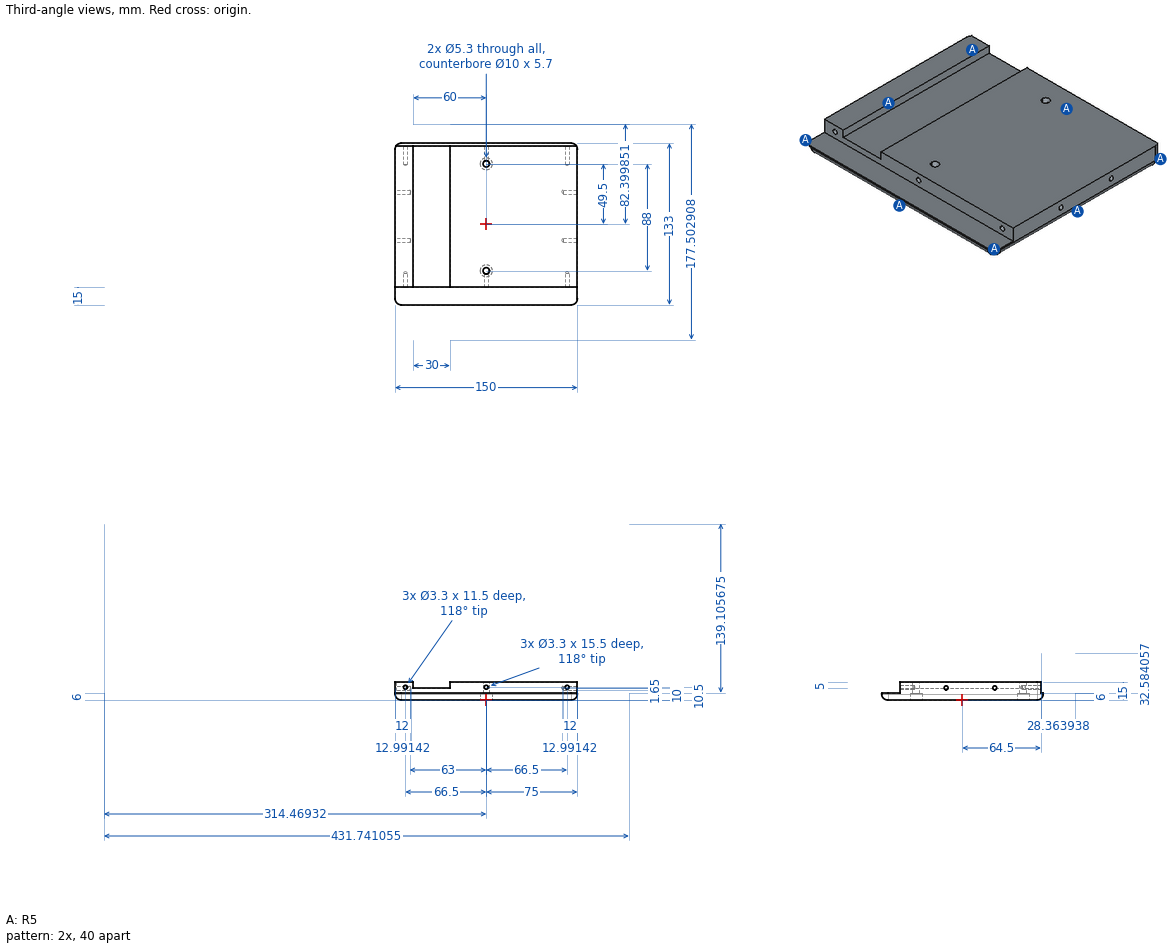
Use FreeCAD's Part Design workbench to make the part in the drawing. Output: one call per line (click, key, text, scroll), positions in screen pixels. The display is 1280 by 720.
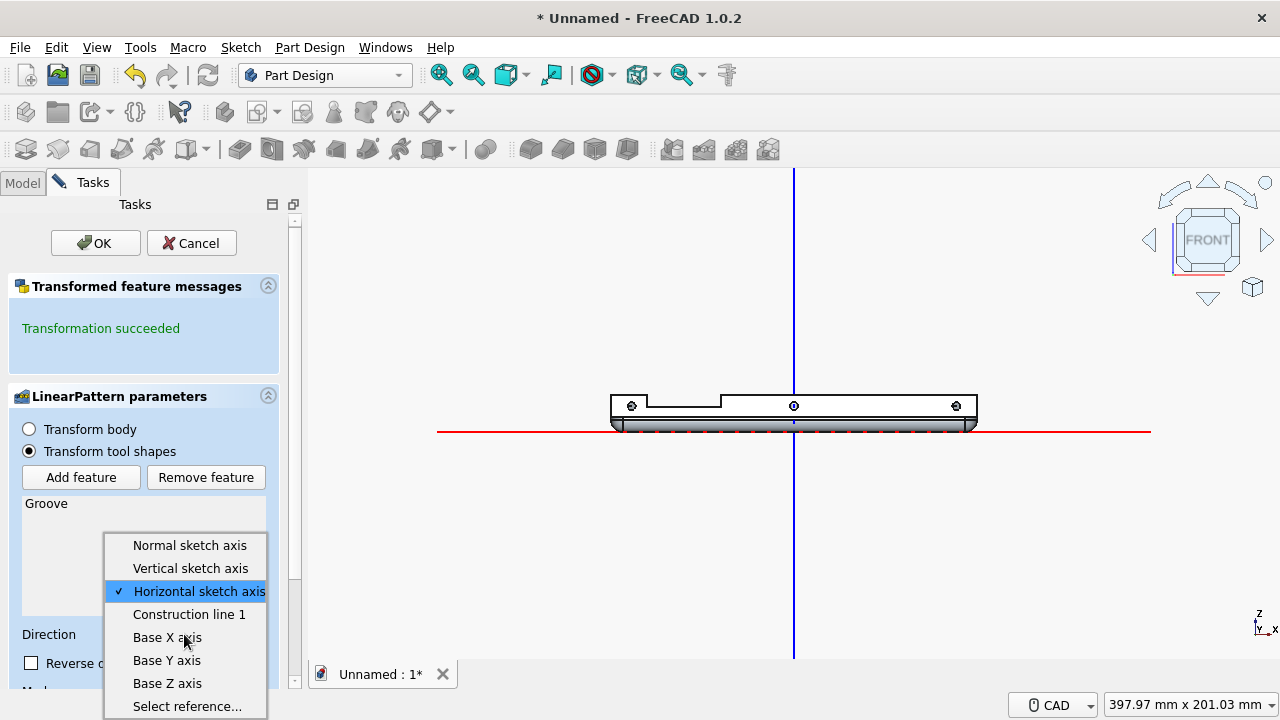
click(184, 660)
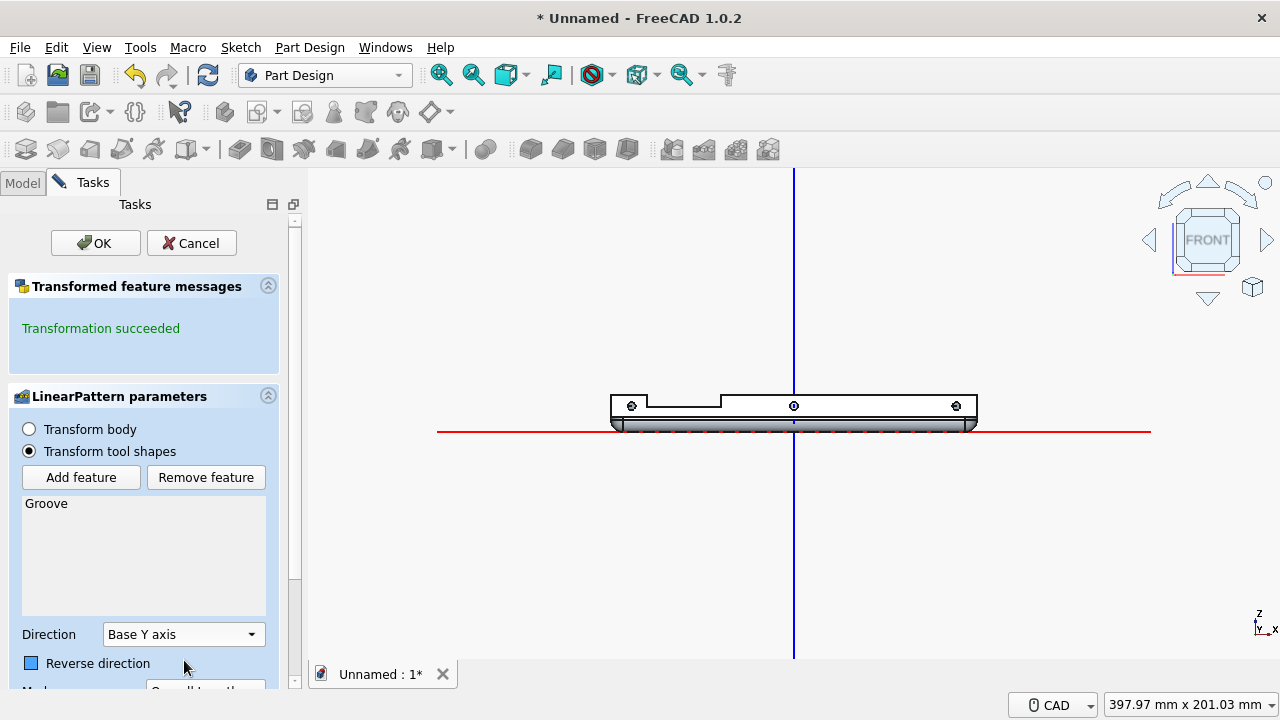
scroll(295, 451, down, 2)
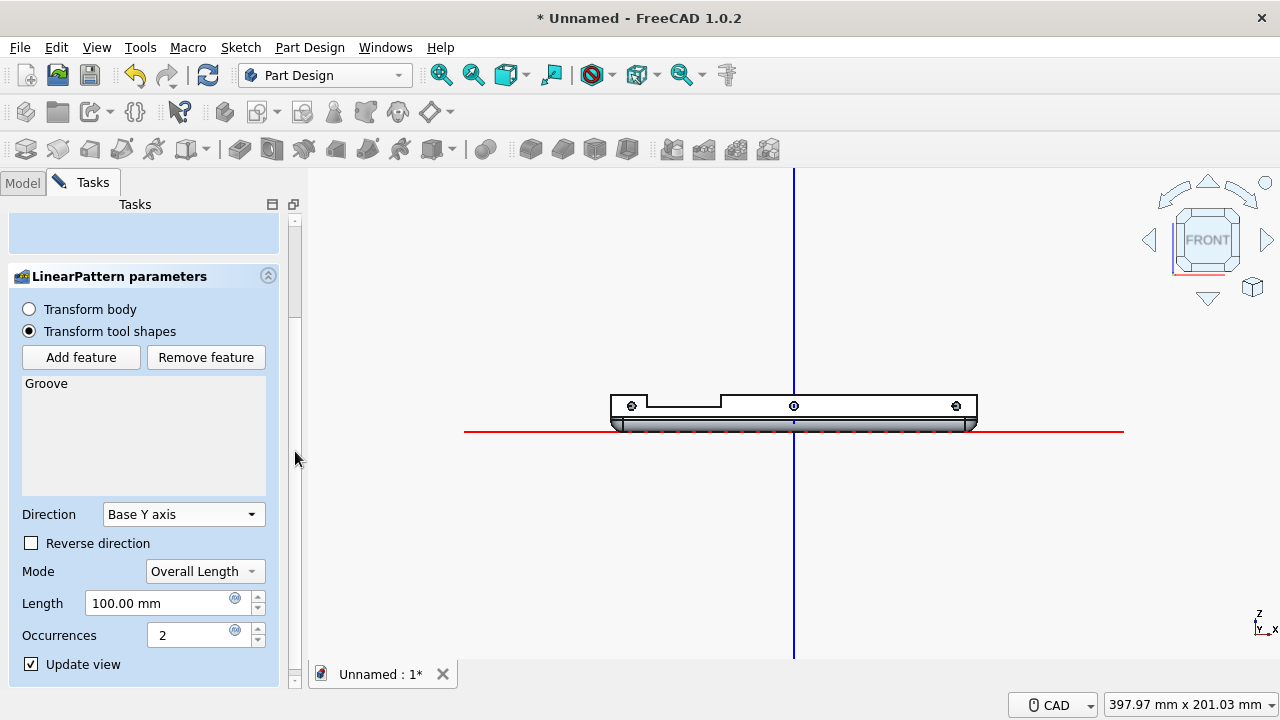
click(206, 572)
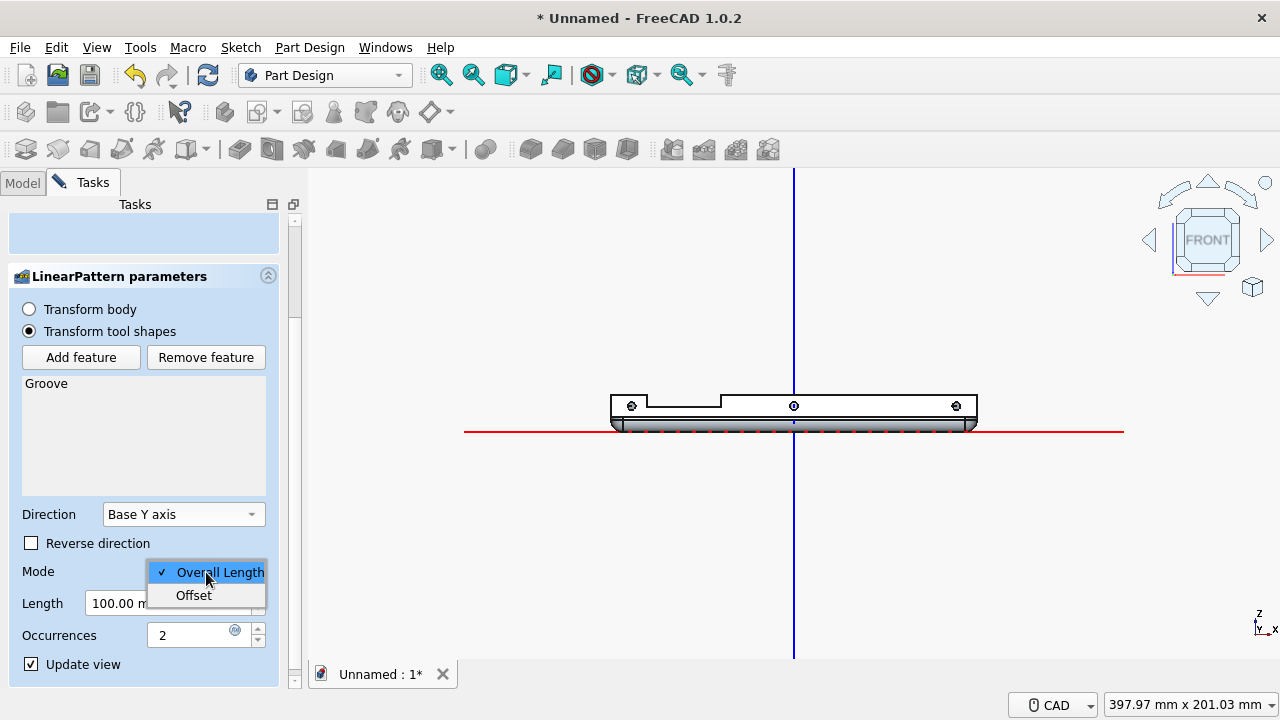
click(206, 596)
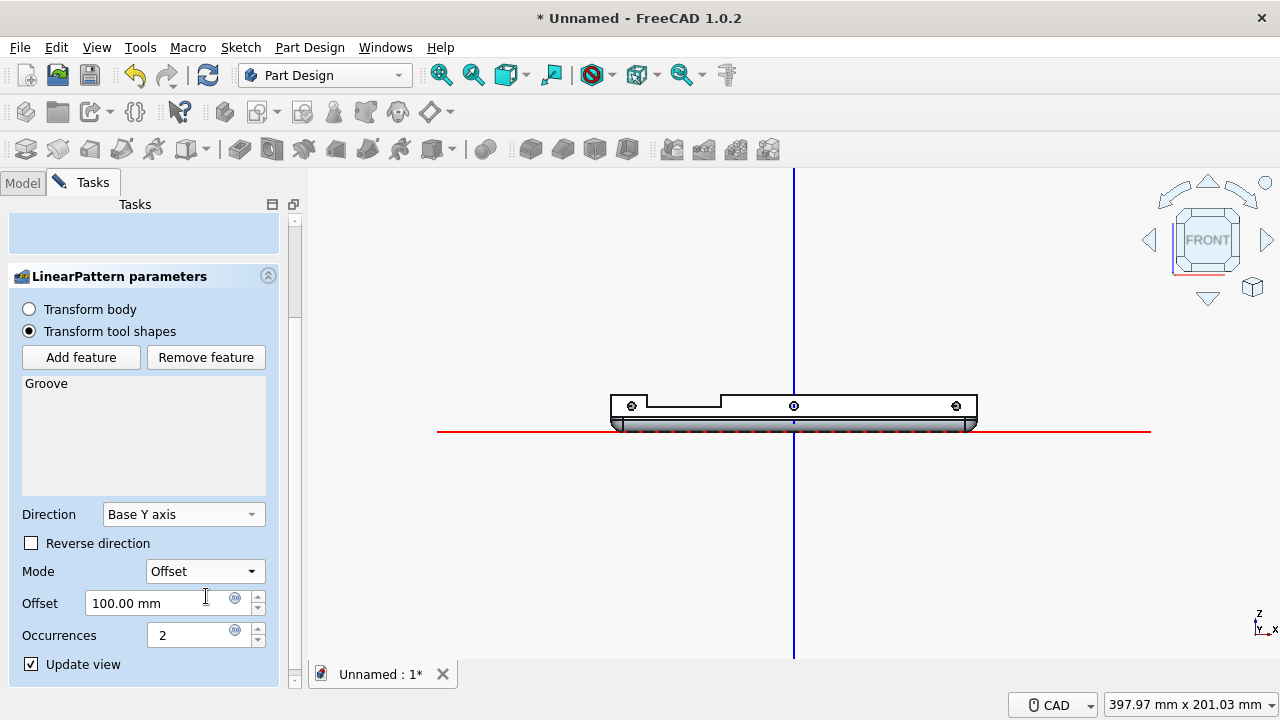
triple_click(168, 603)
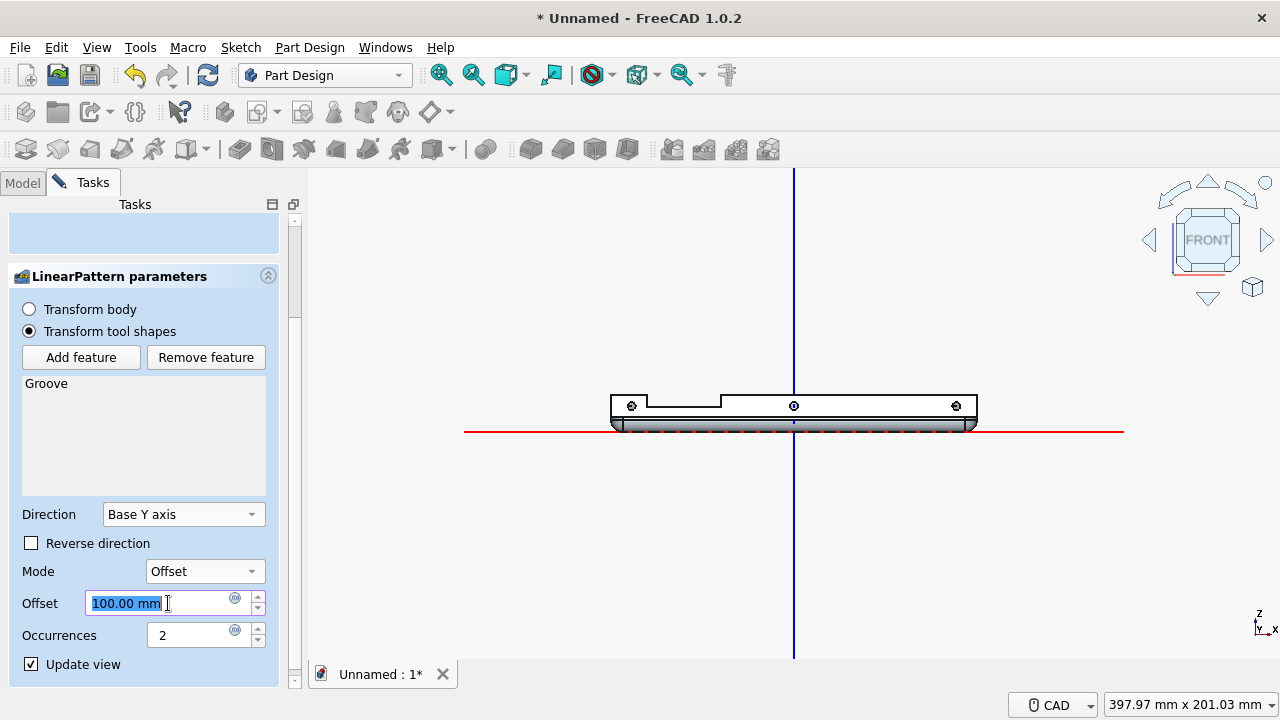
text(40)
key(Tab)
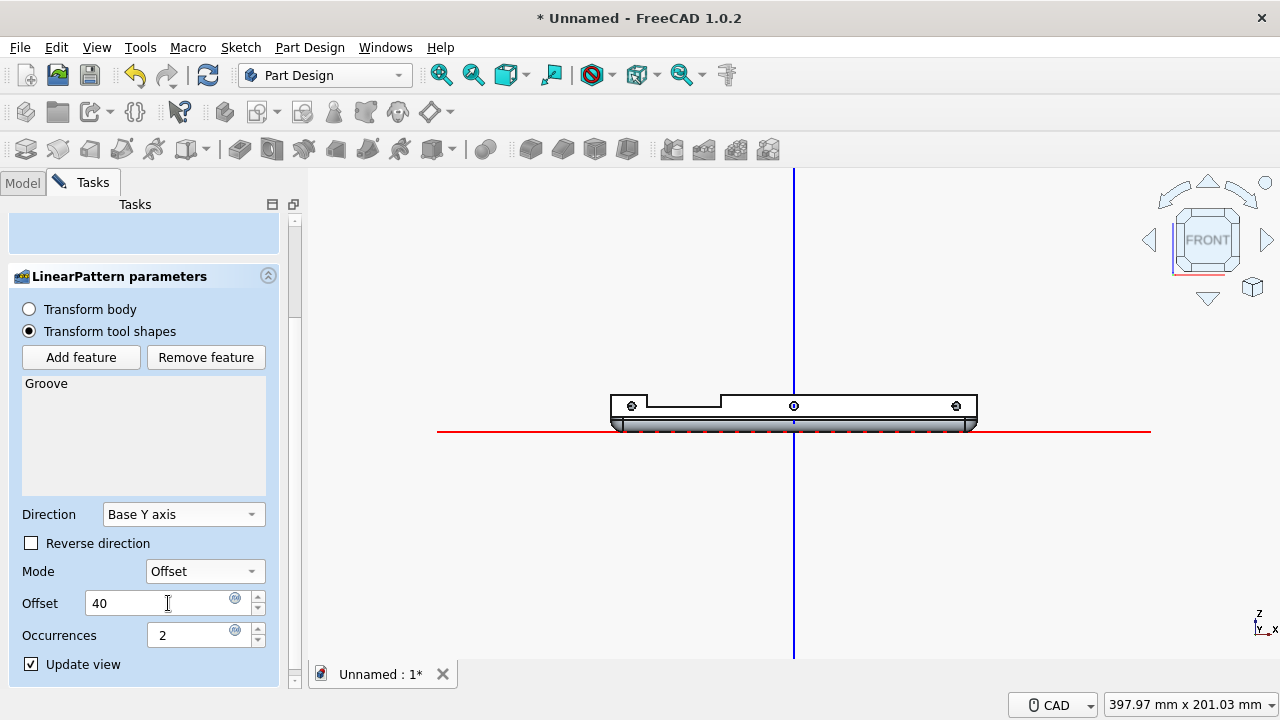
triple_click(198, 635)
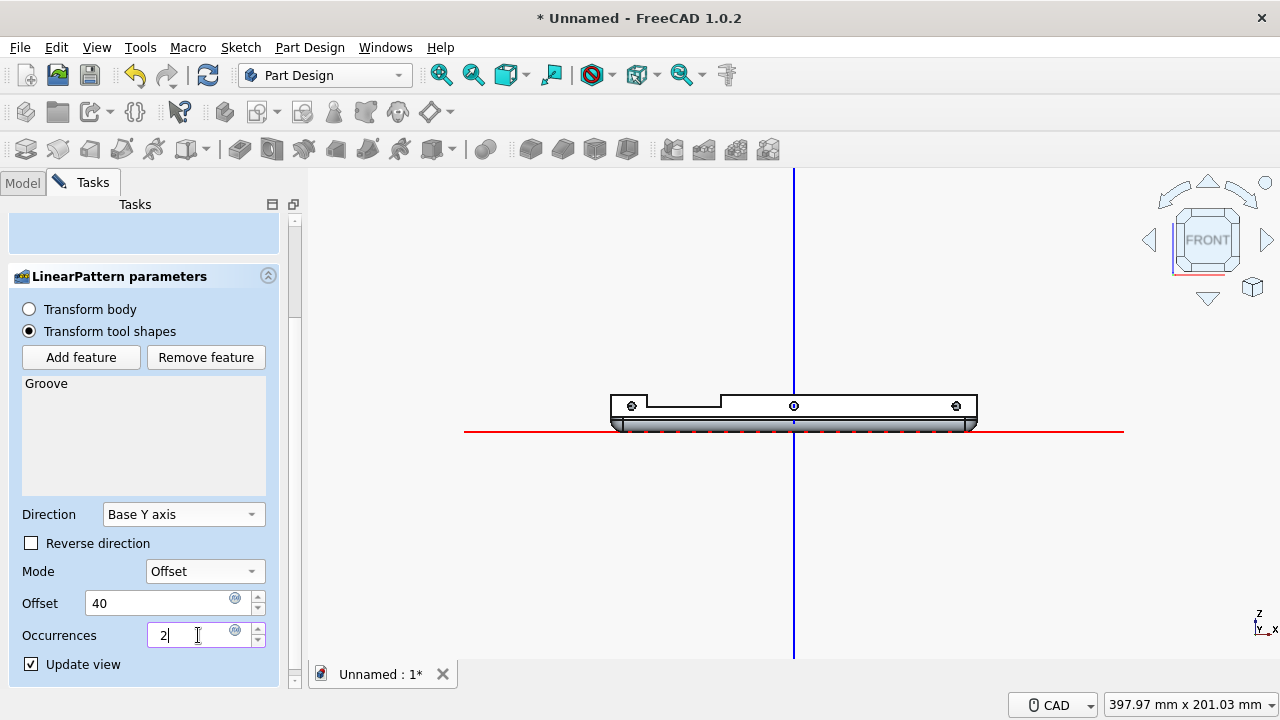
text(2)
key(Tab)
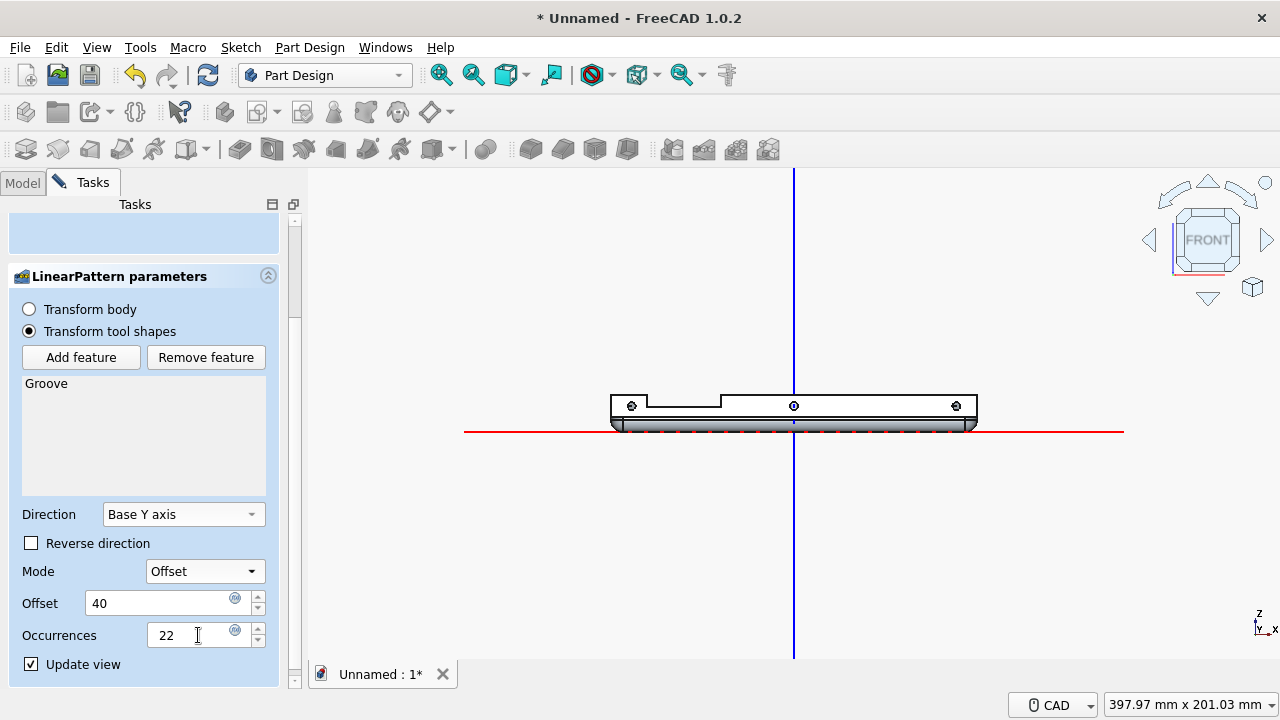
click(30, 543)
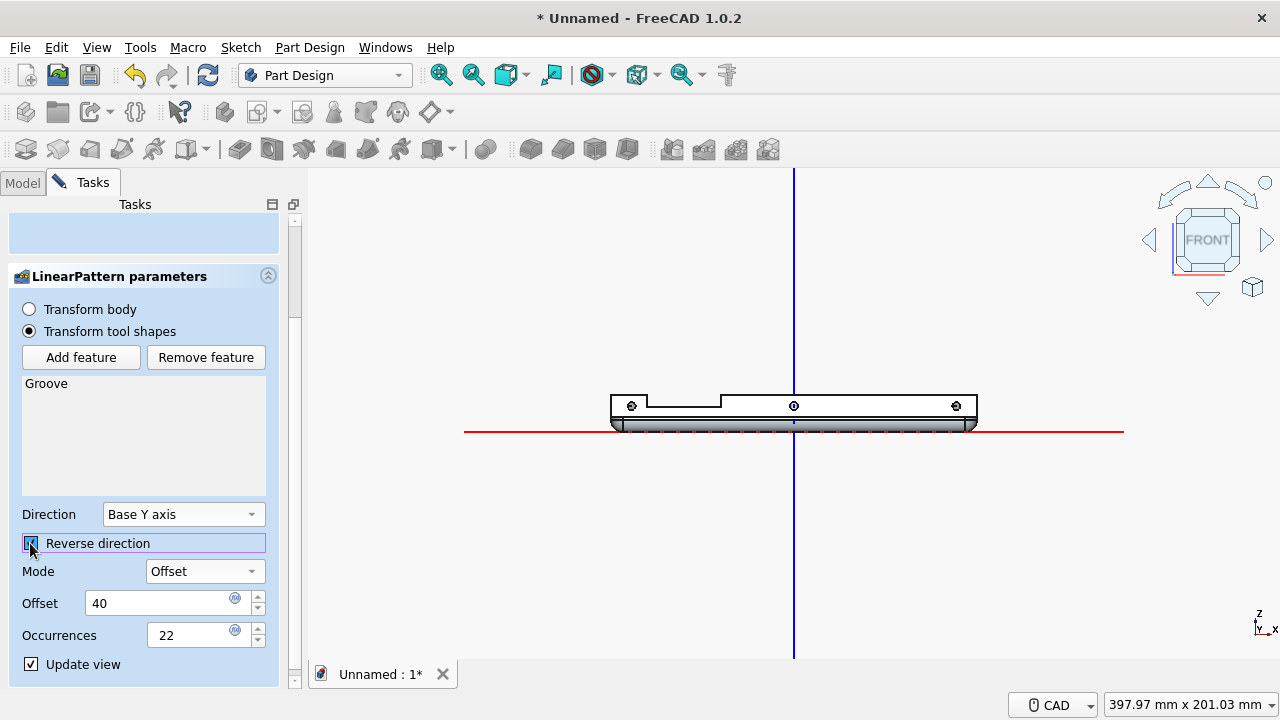
scroll(295, 451, up, 3)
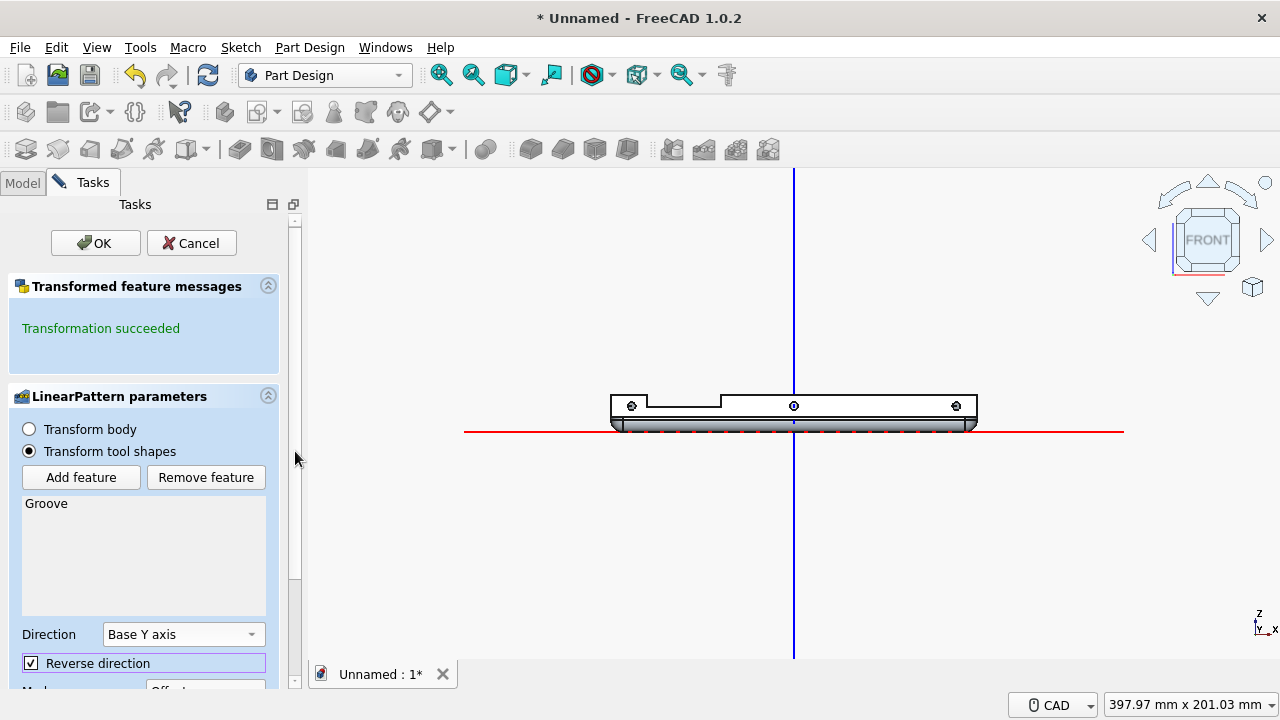
click(96, 243)